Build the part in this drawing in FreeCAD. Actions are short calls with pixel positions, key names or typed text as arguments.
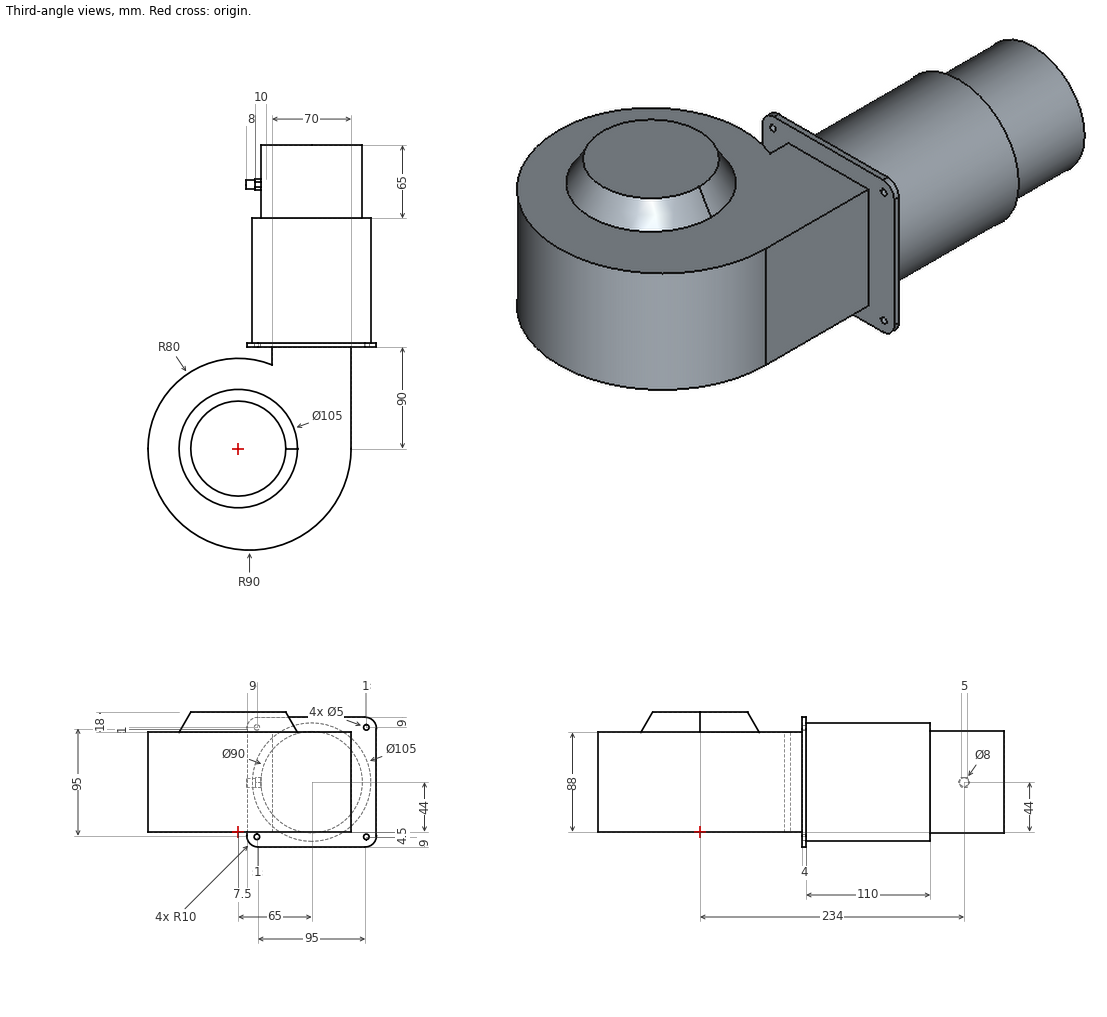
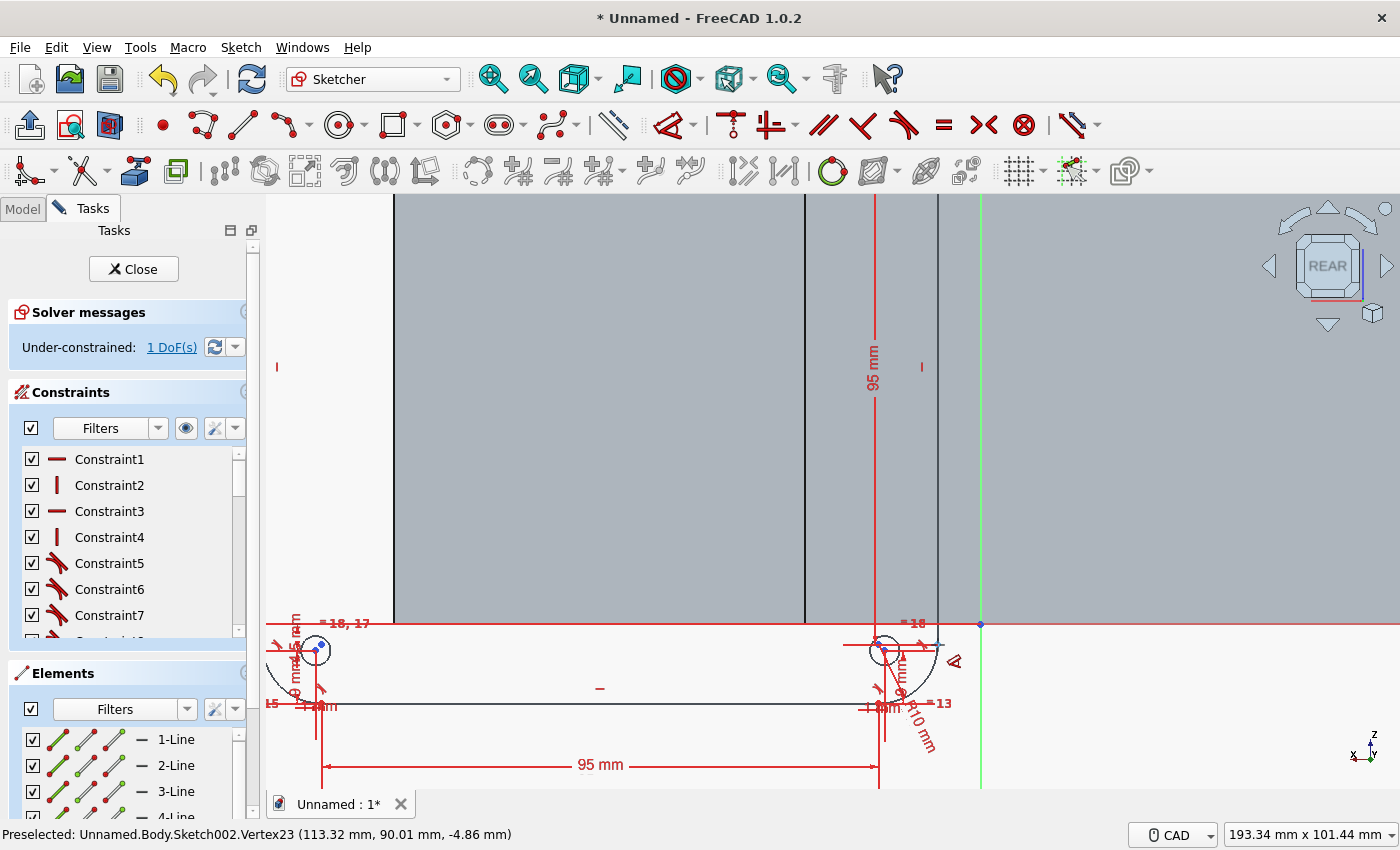
click(938, 645)
click(959, 590)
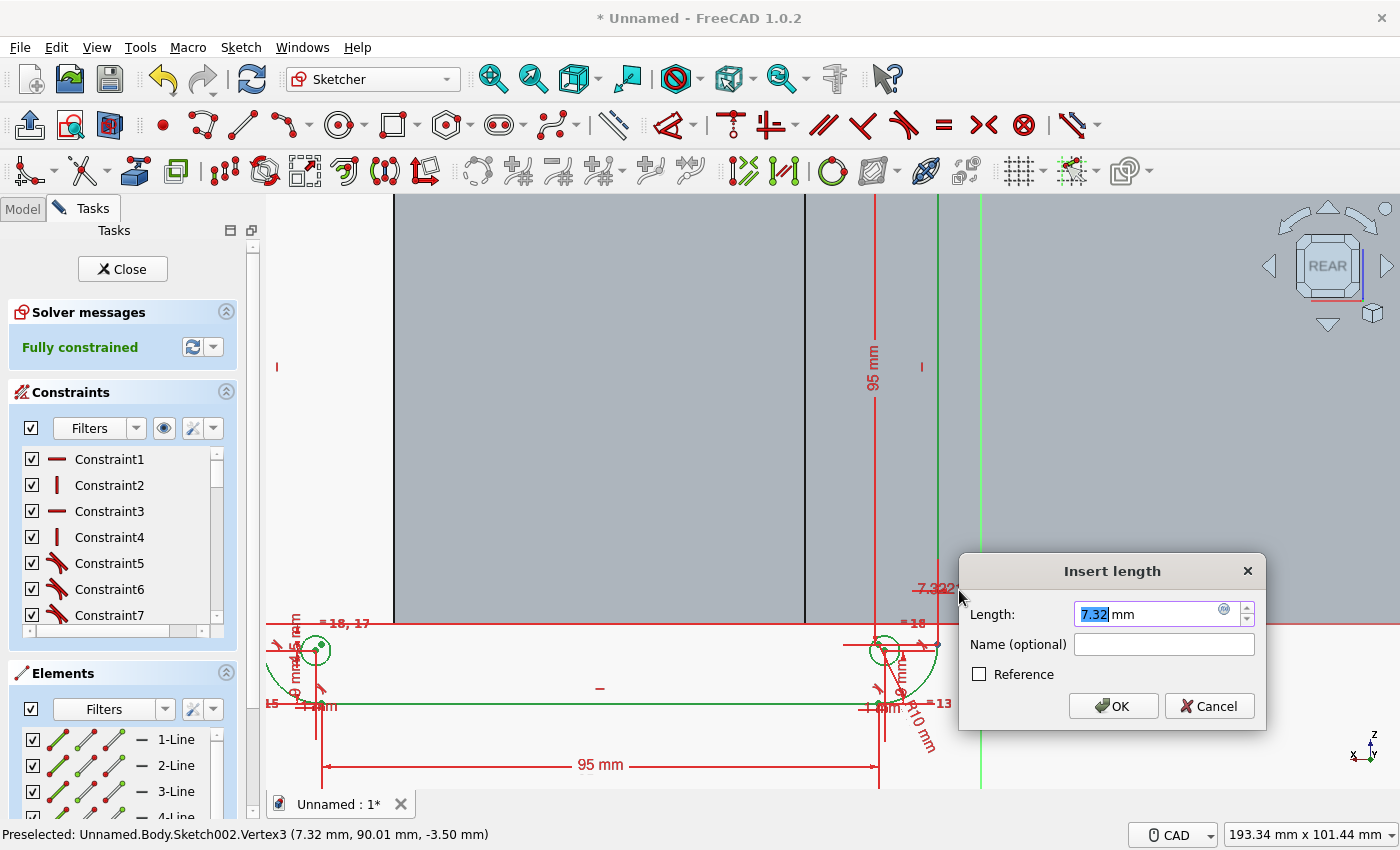
text(7.5)
key(Return)
key(Escape)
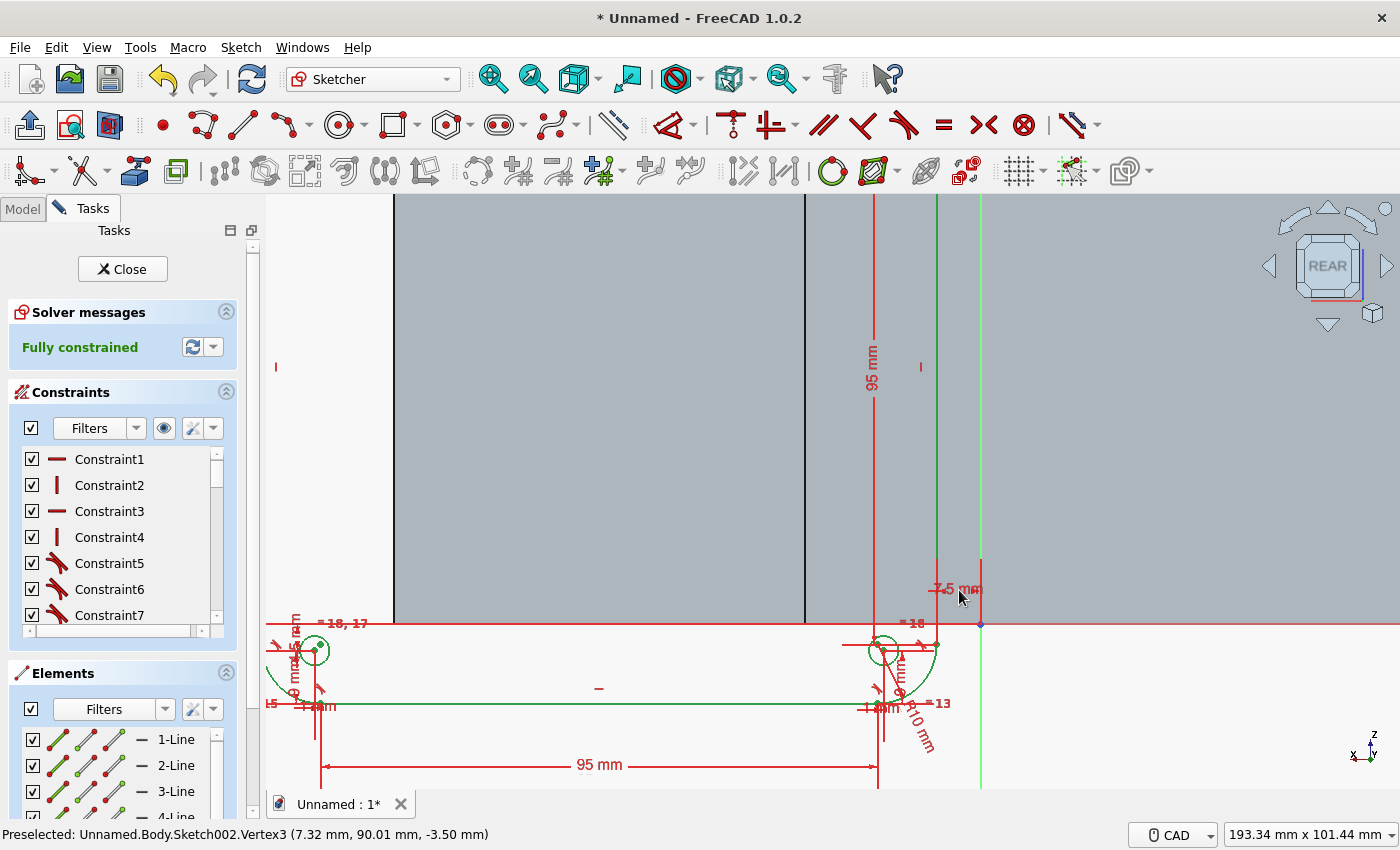
click(123, 269)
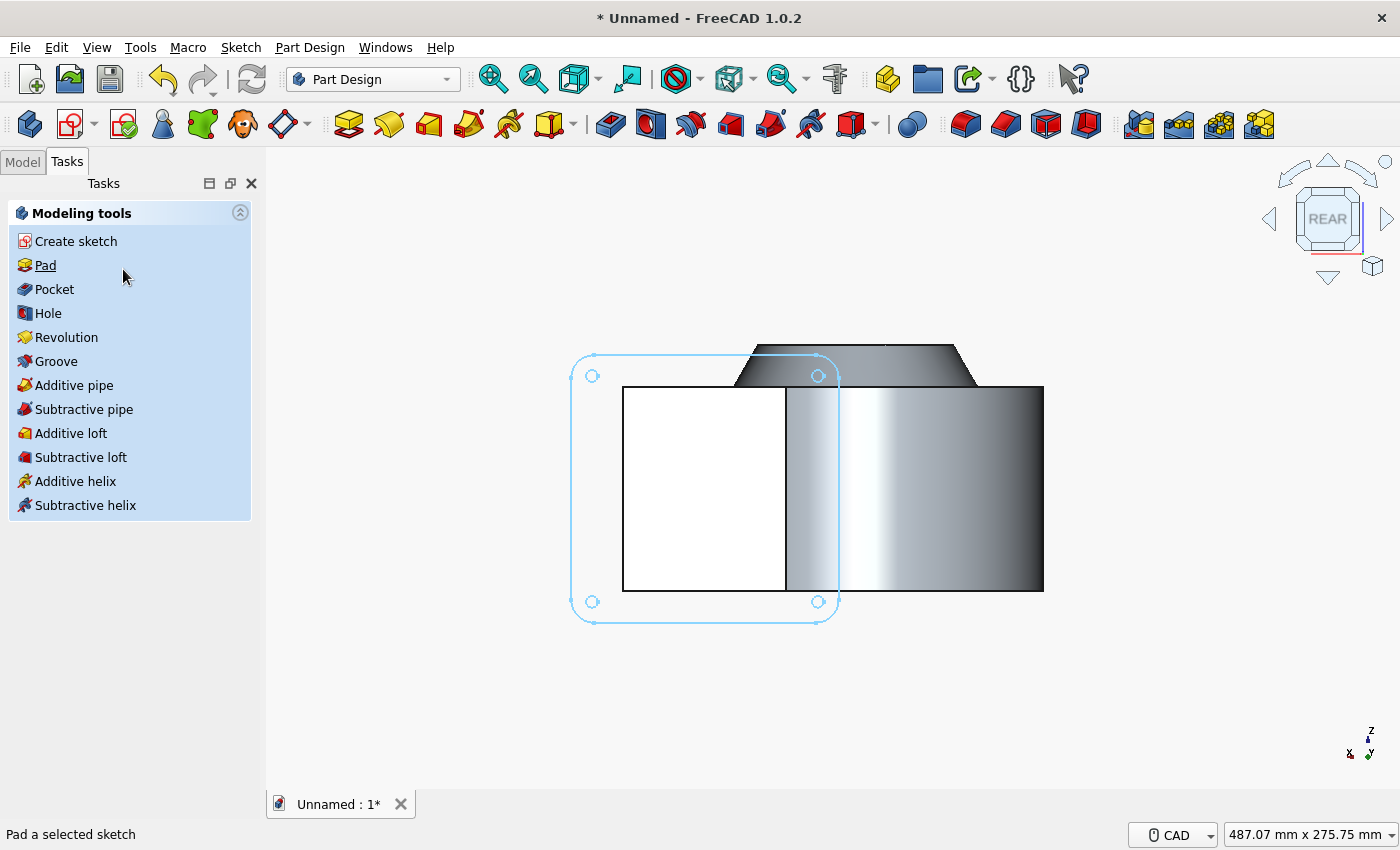
click(350, 124)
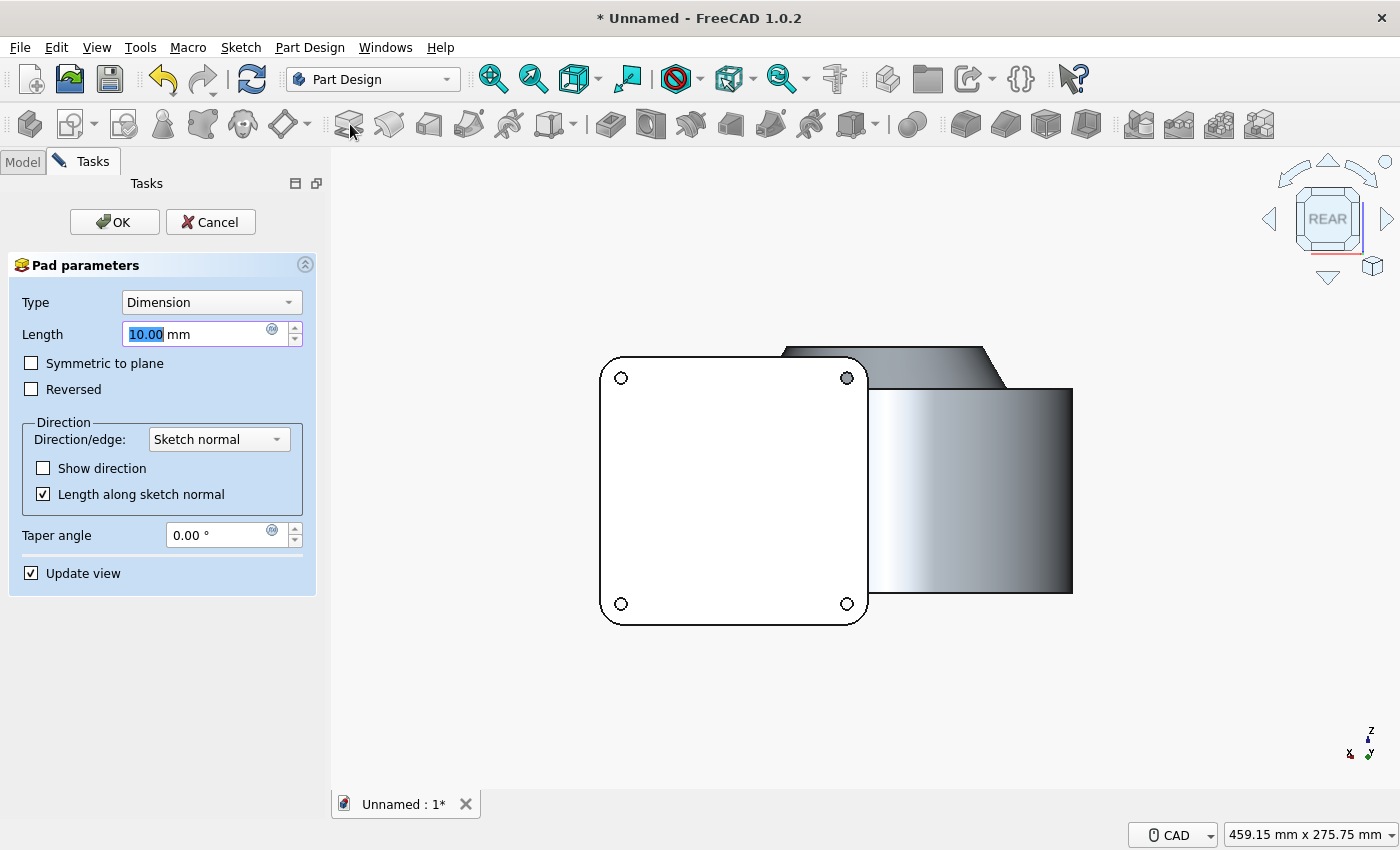
text(4)
key(Tab)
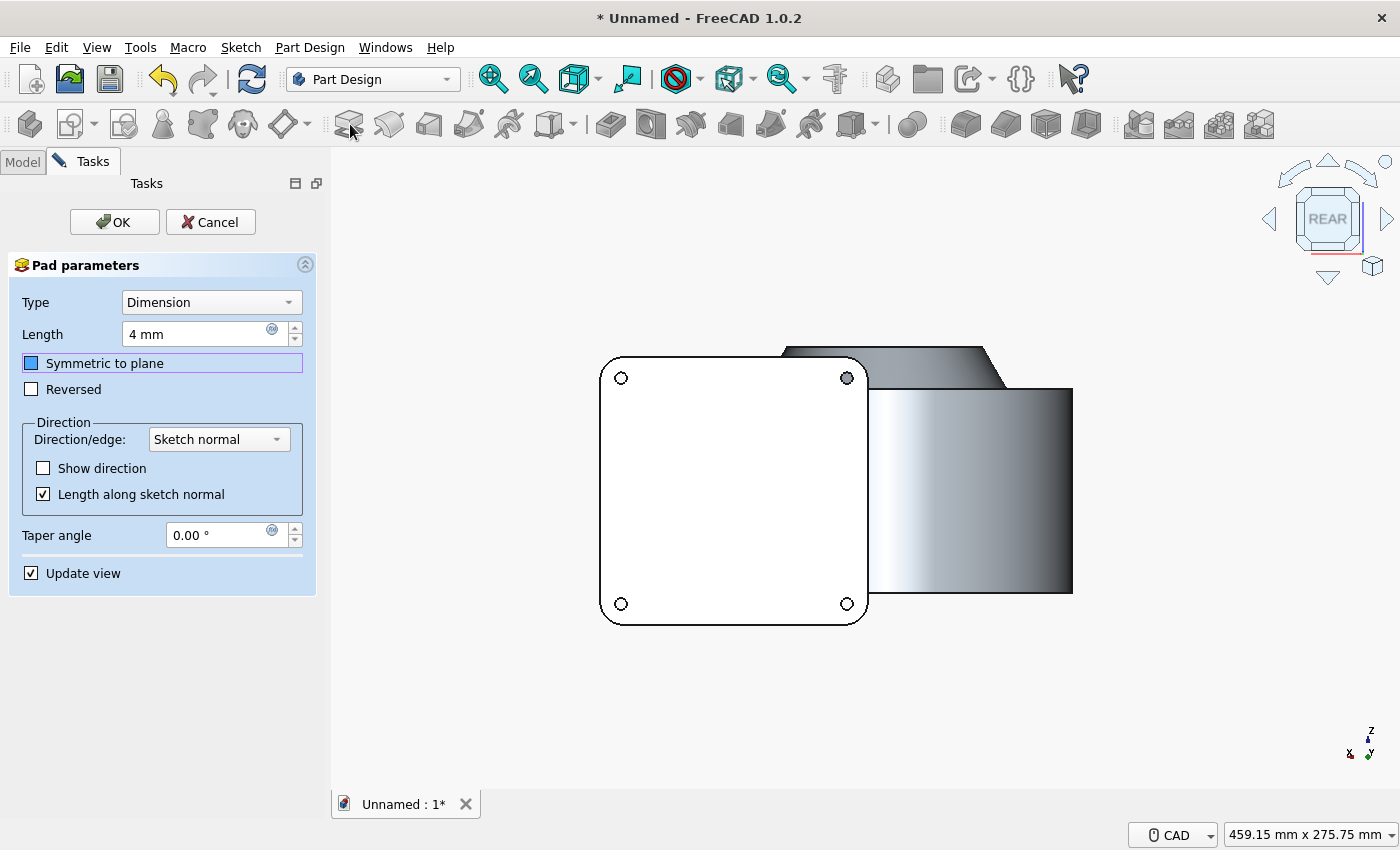
click(115, 222)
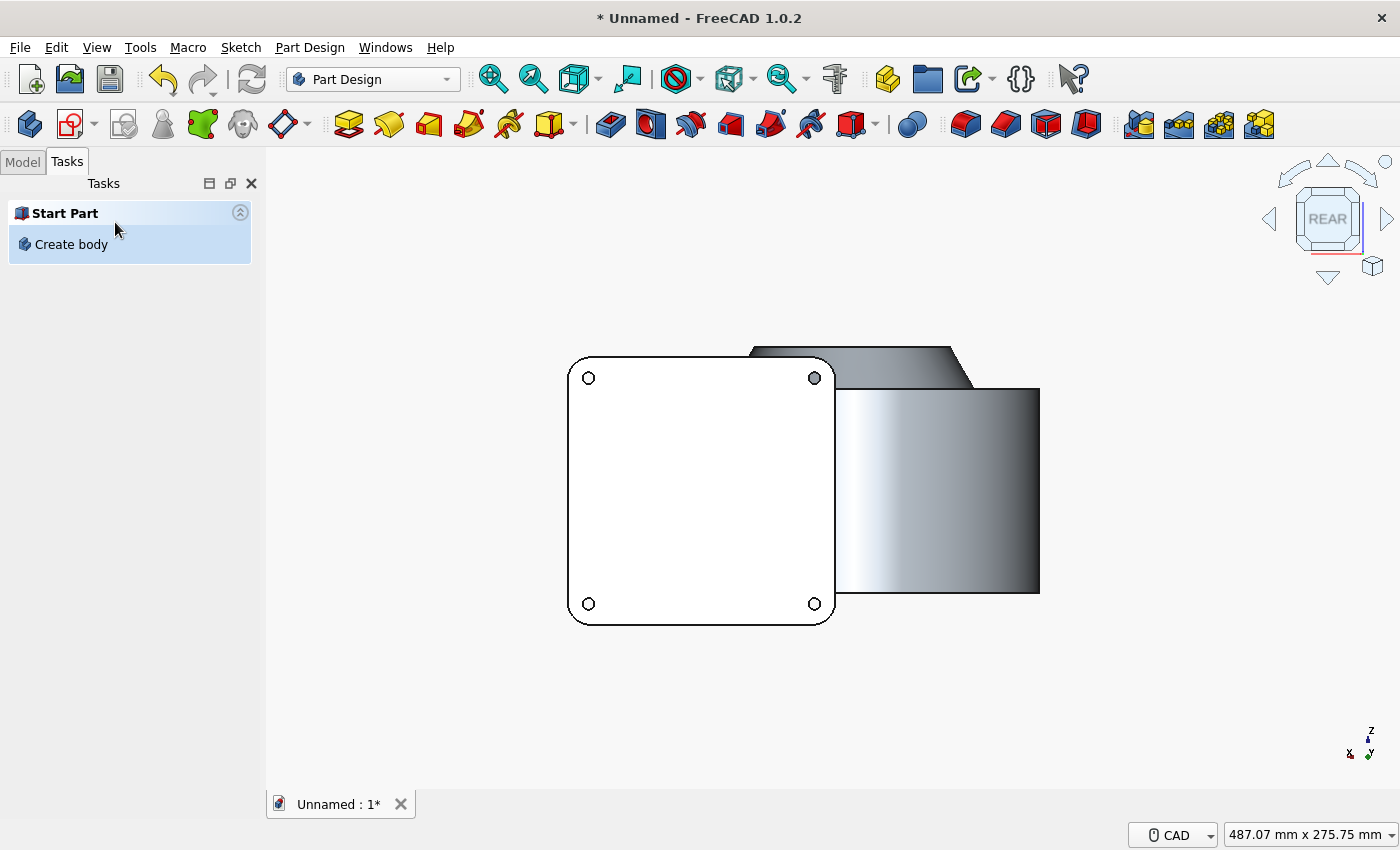
click(494, 80)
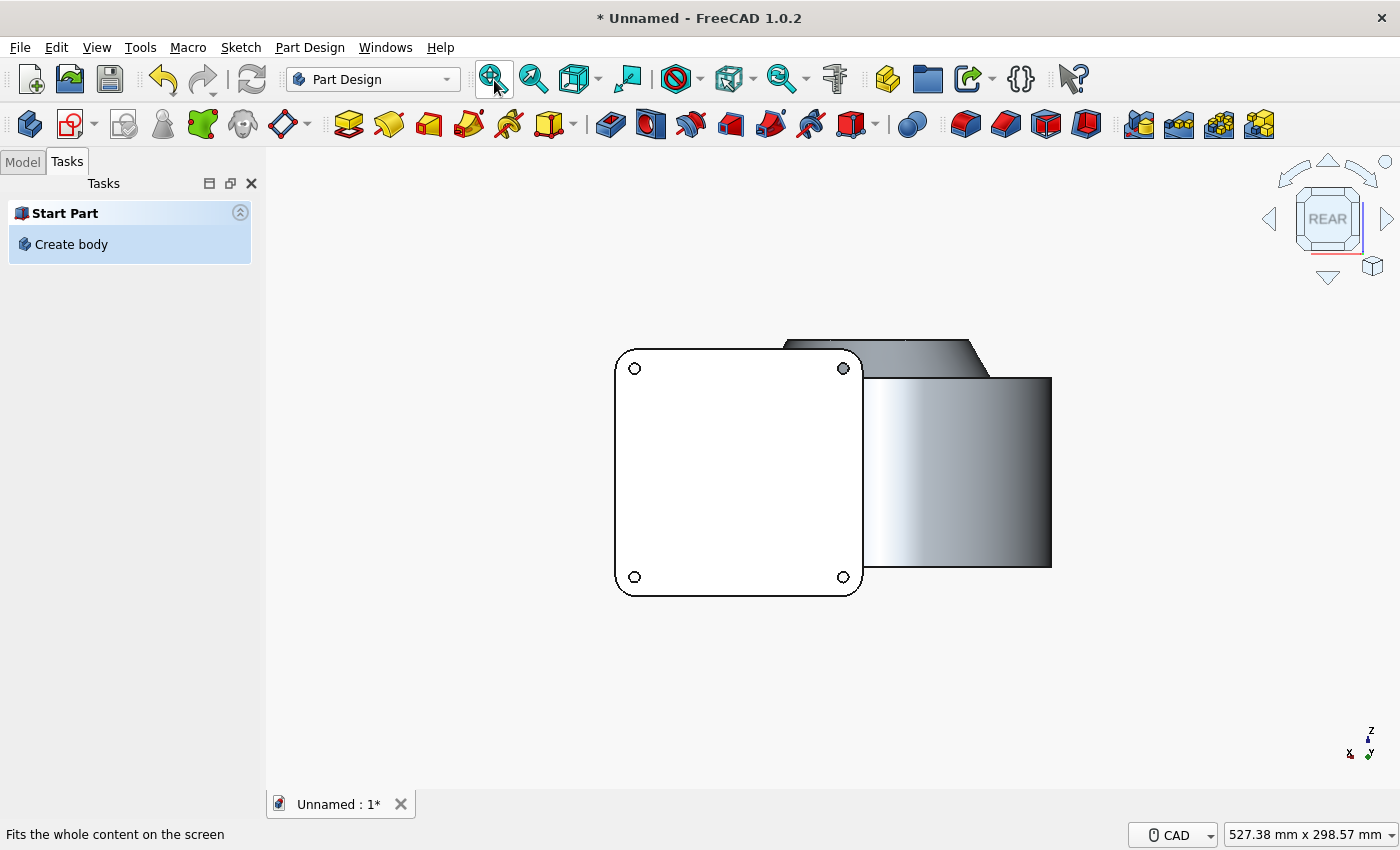
click(739, 472)